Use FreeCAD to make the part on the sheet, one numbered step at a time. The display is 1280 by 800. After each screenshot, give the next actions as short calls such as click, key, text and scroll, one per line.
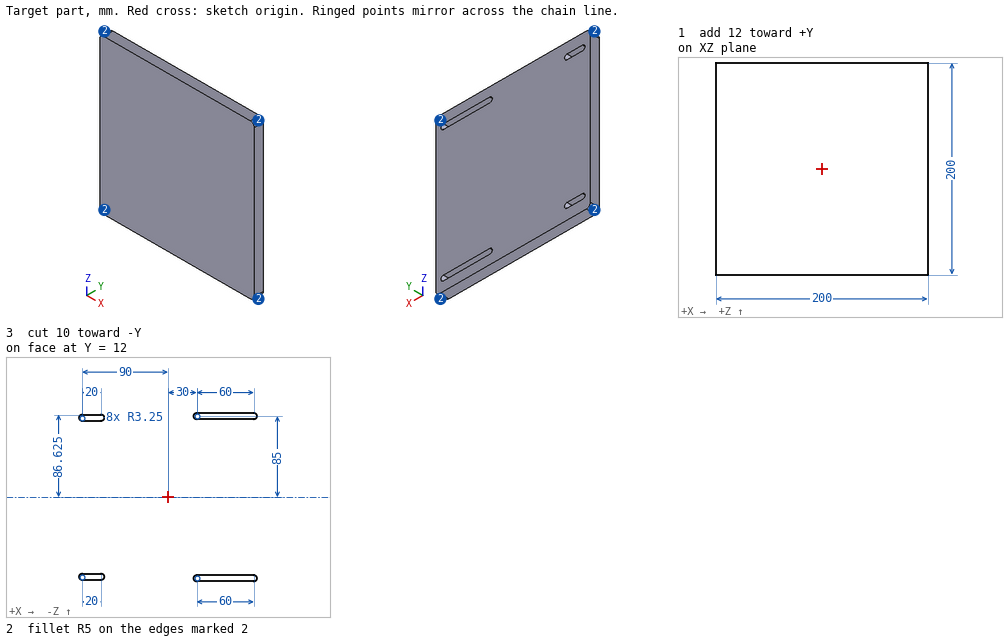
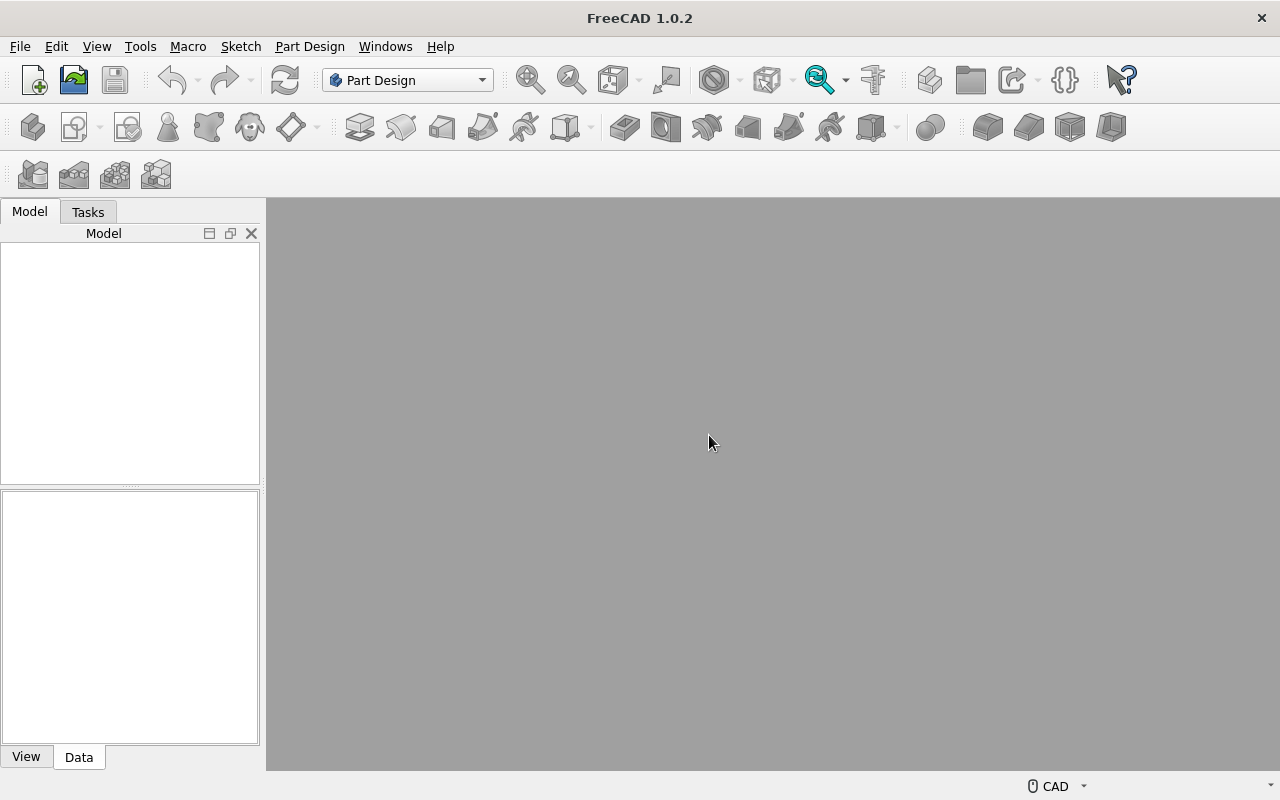
click(33, 80)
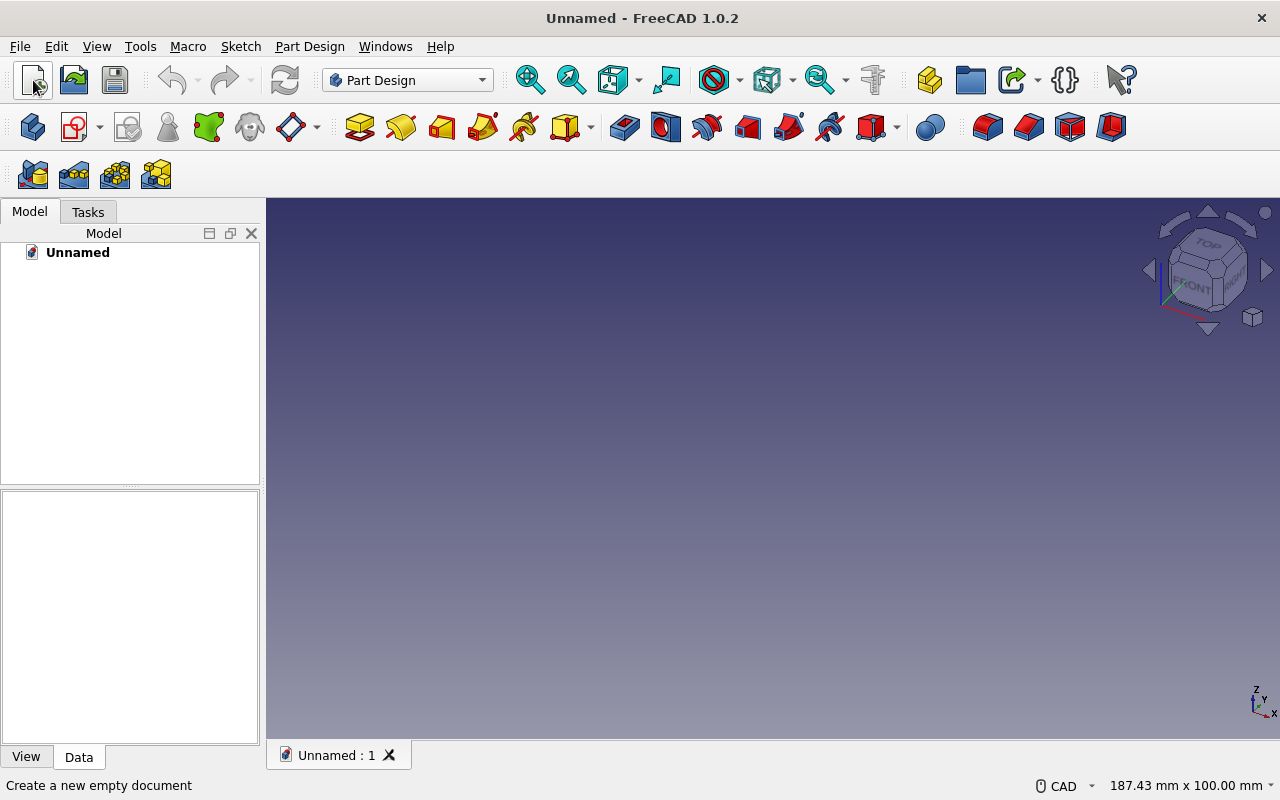
click(74, 128)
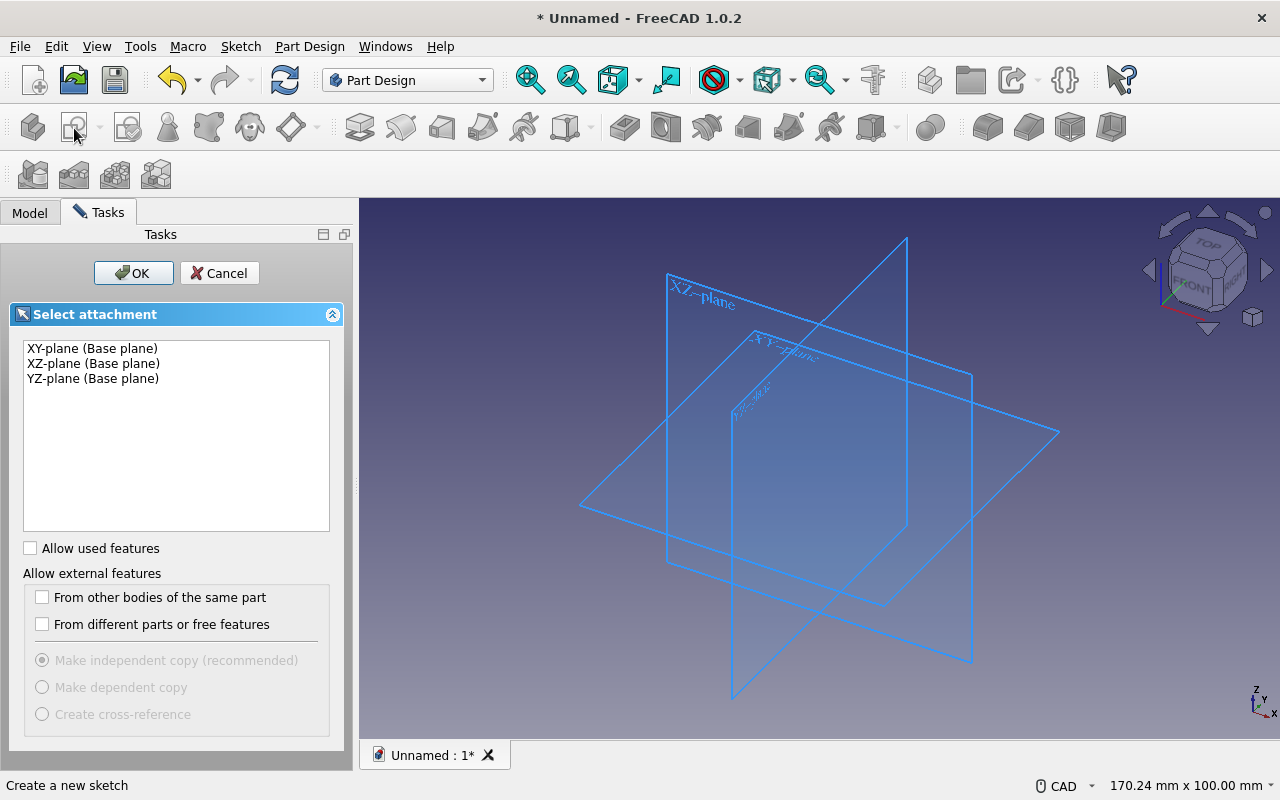
click(84, 364)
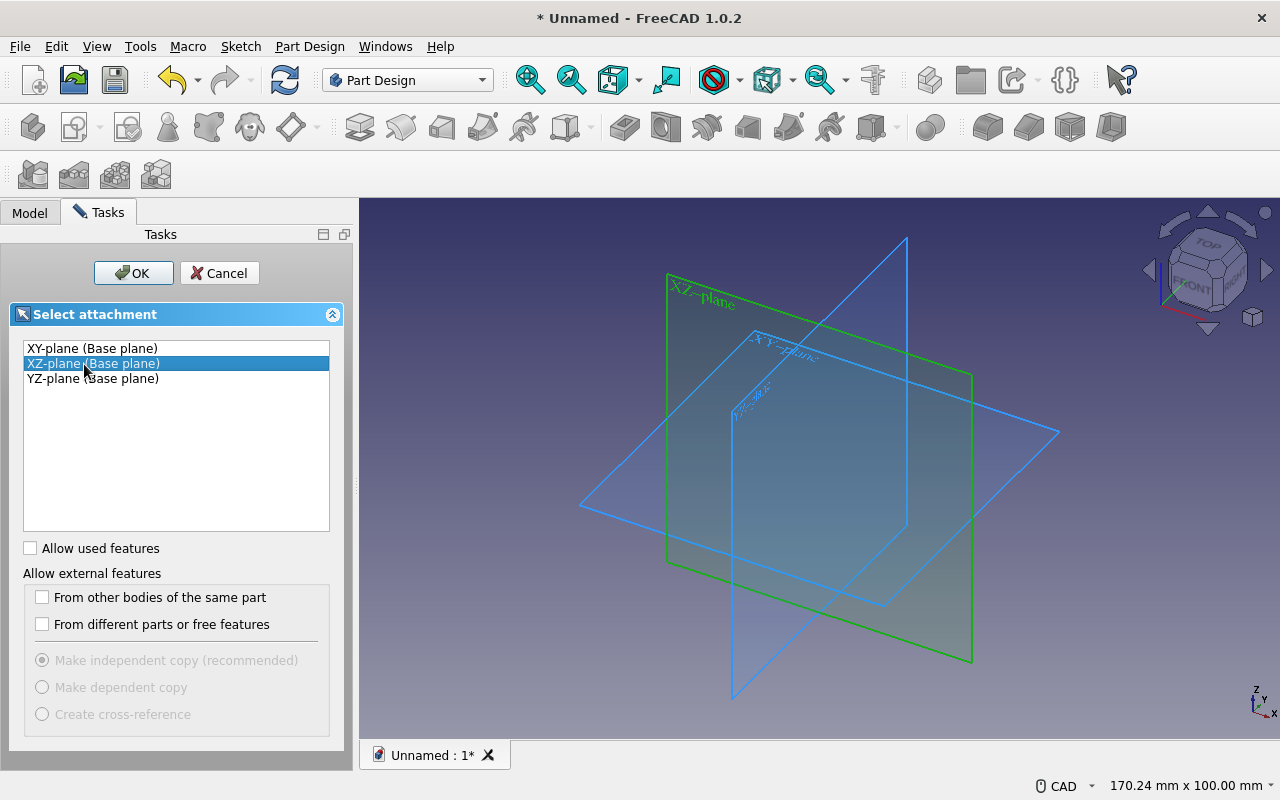
click(134, 273)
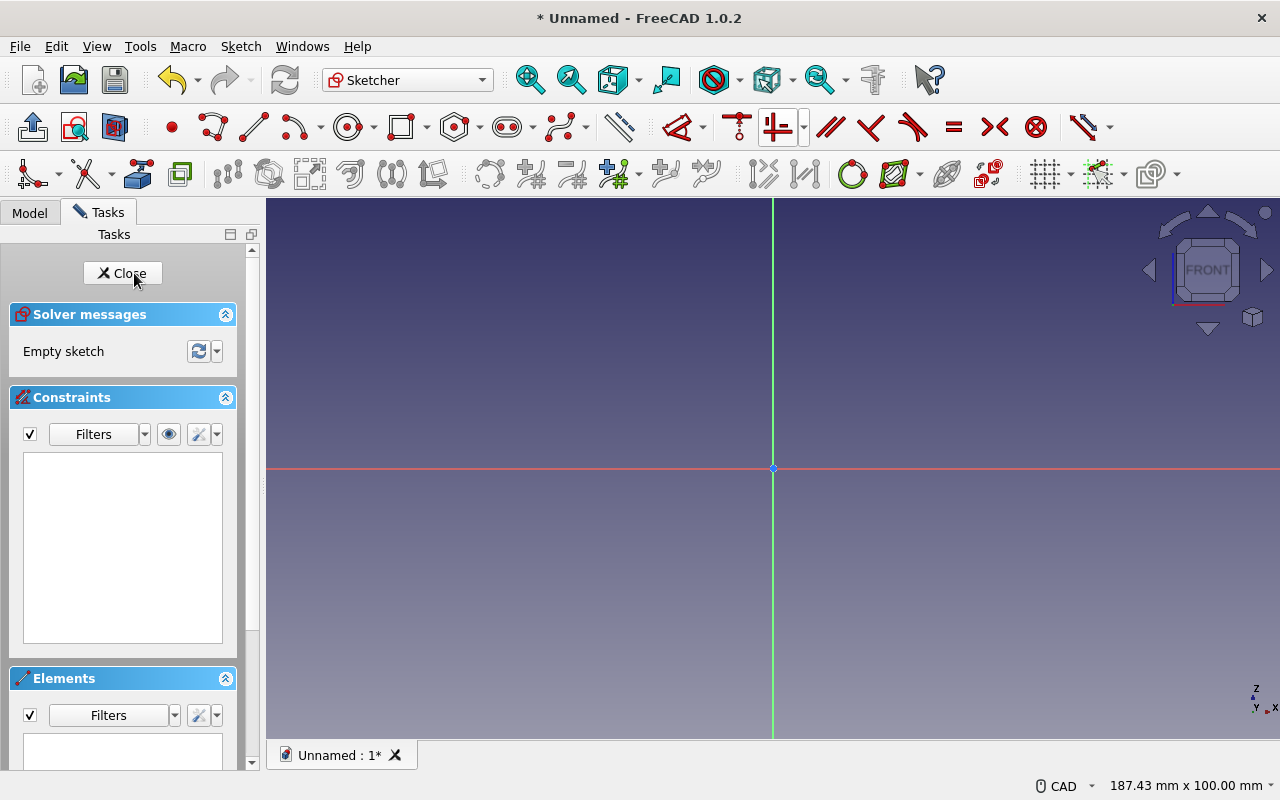
scroll(675, 468, down, 6)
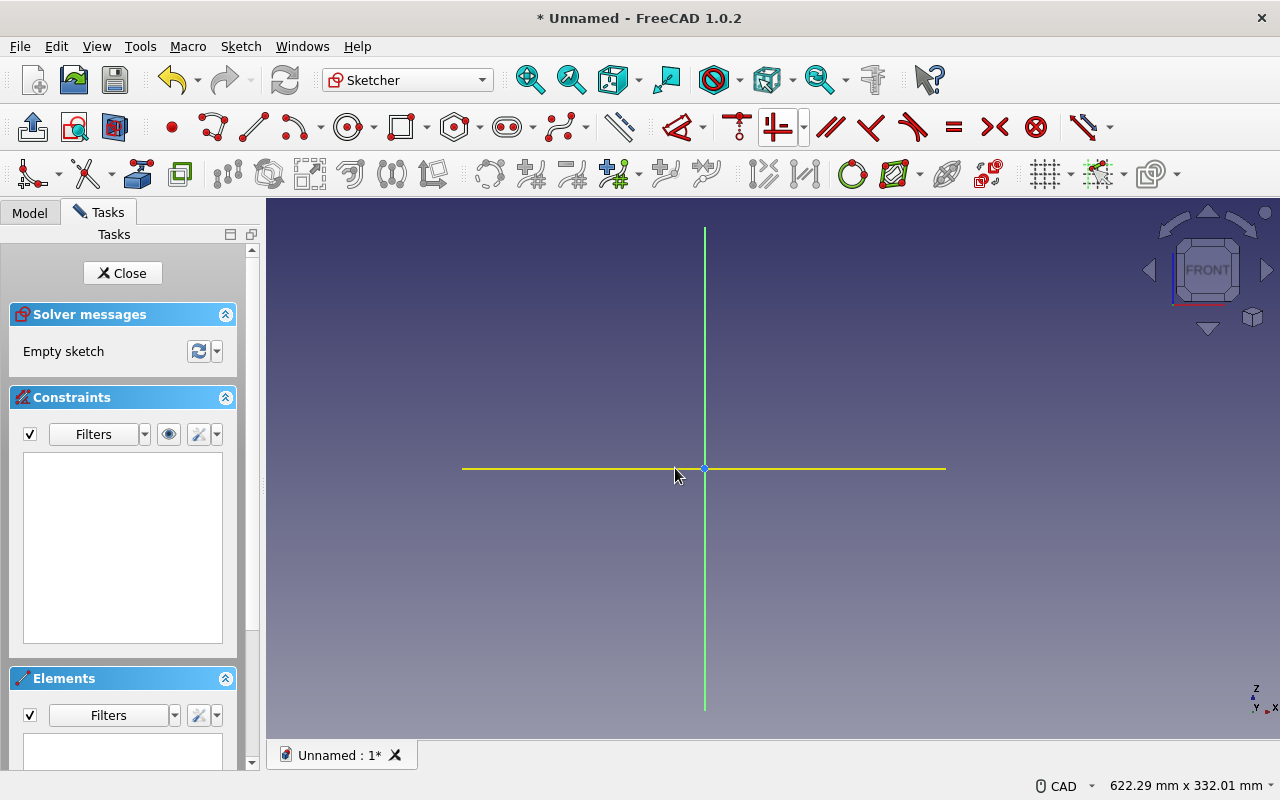
click(426, 128)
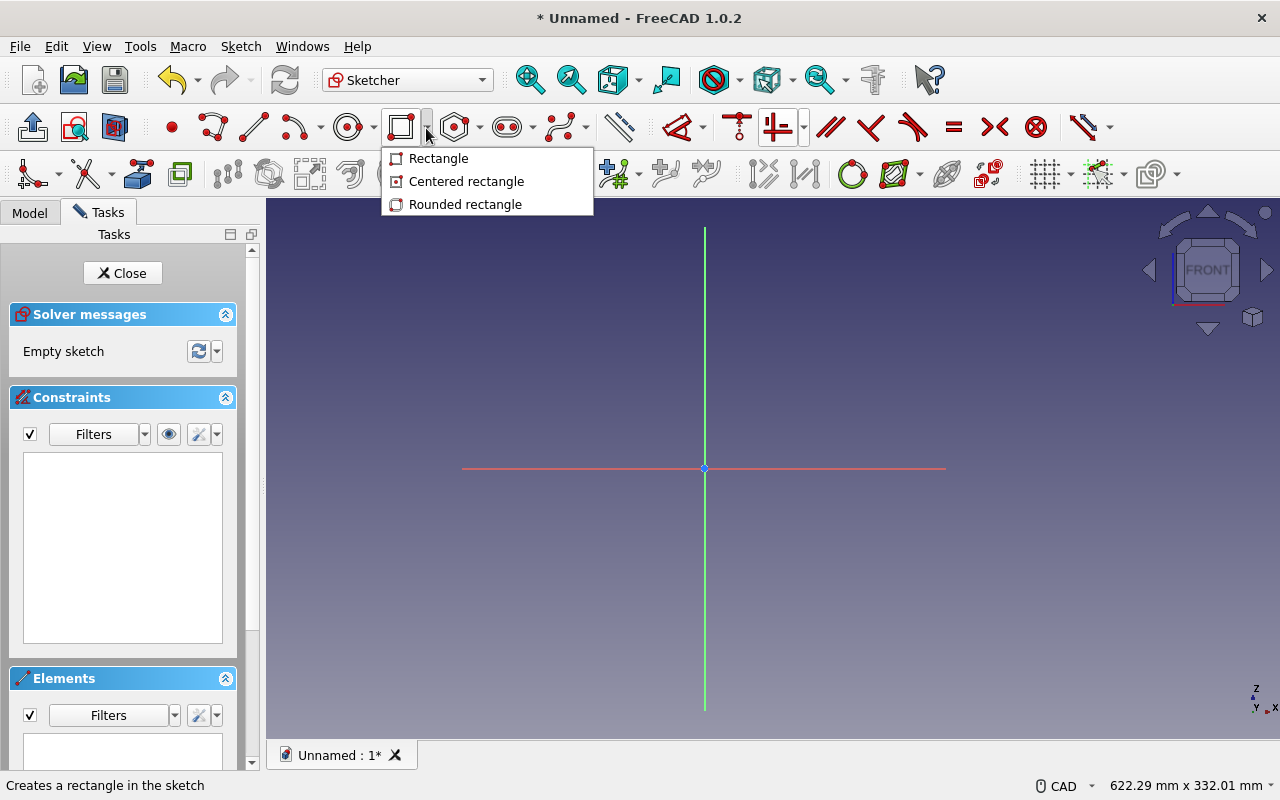
click(488, 182)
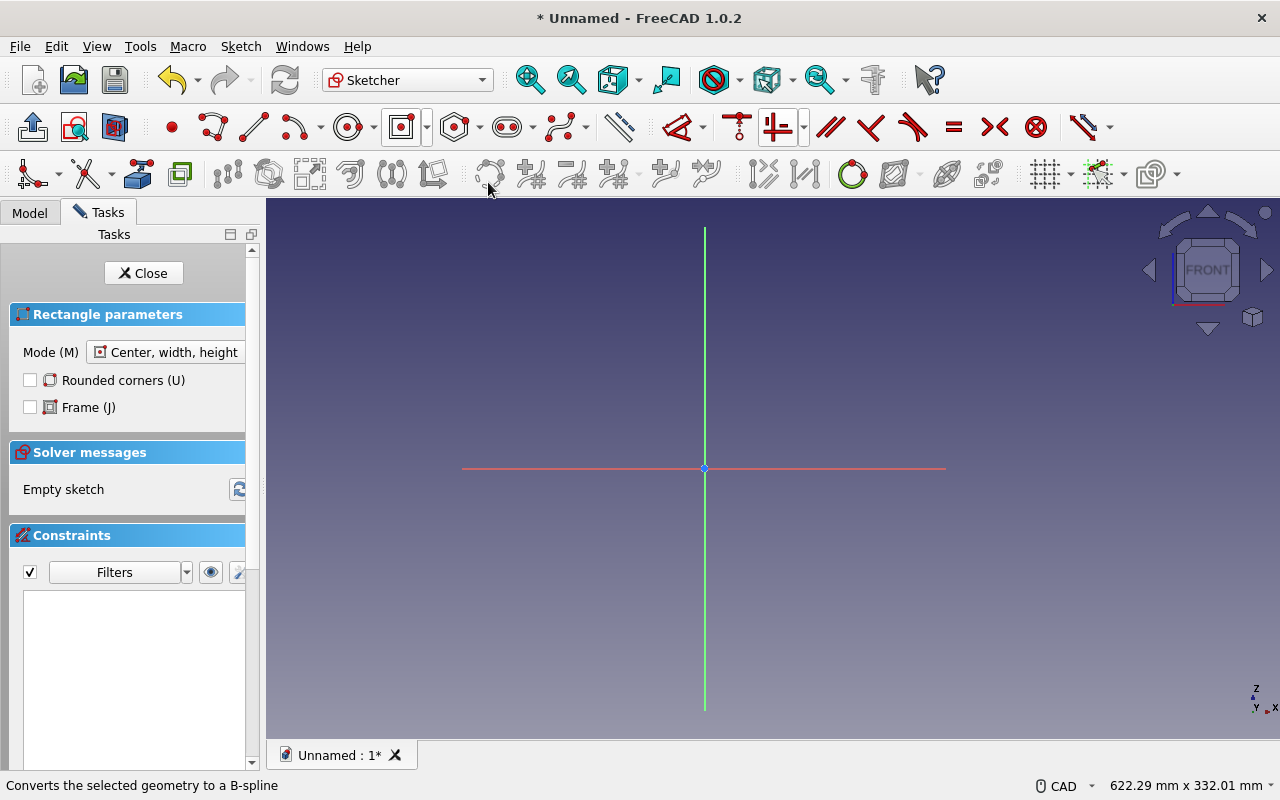
click(705, 468)
click(868, 306)
key(Escape)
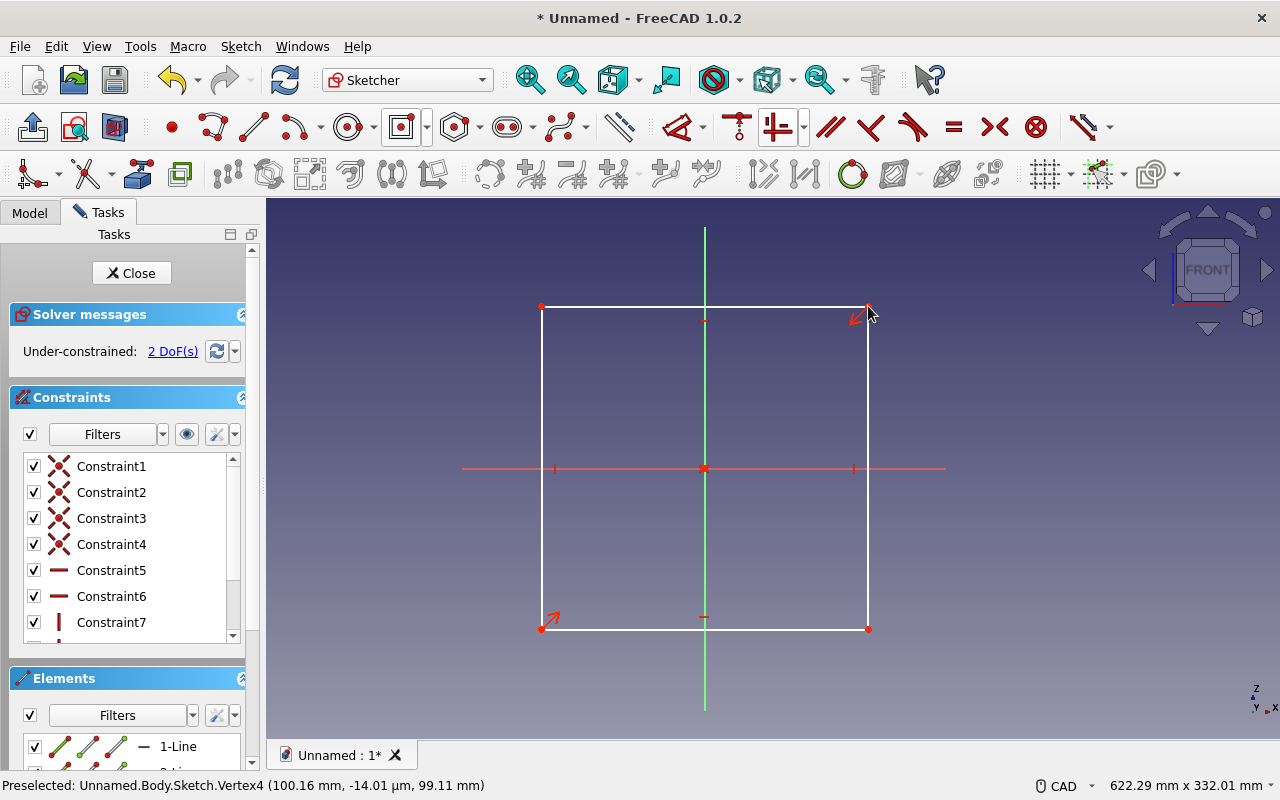
click(676, 128)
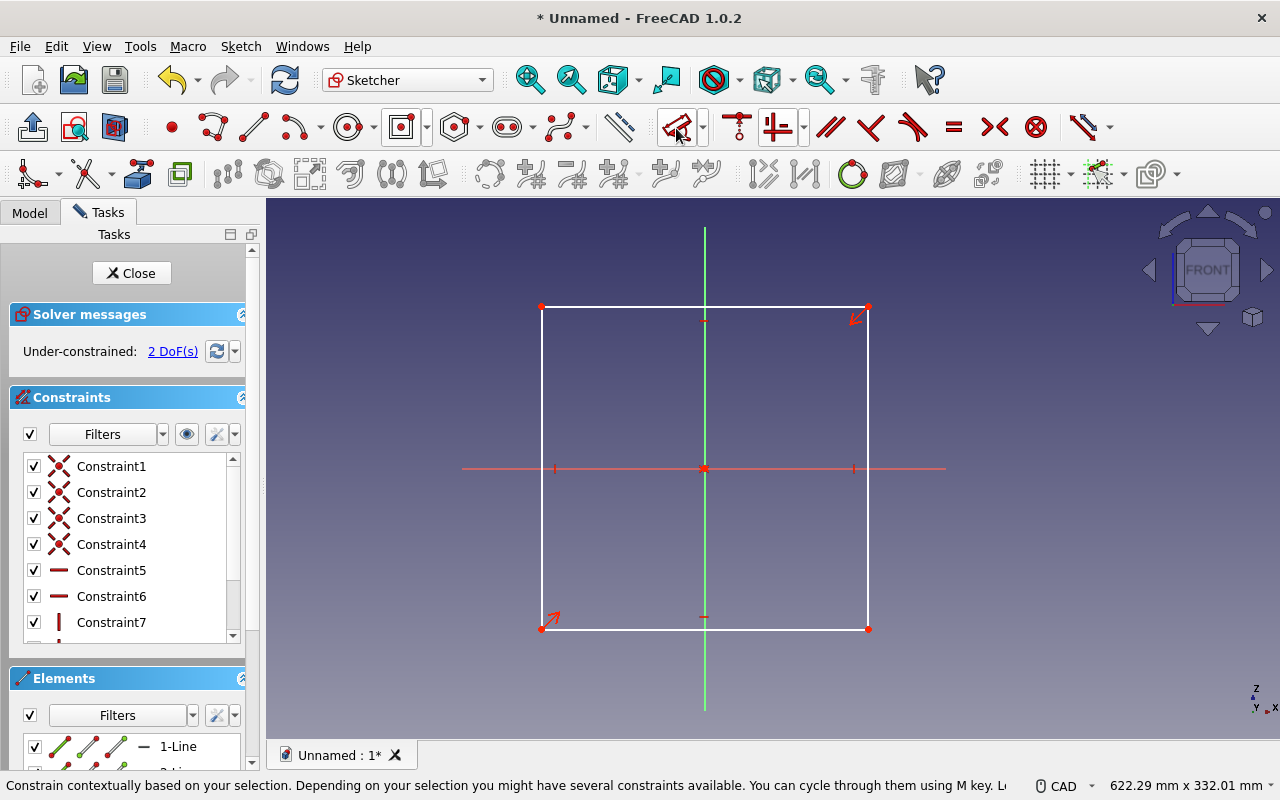
click(640, 630)
click(630, 664)